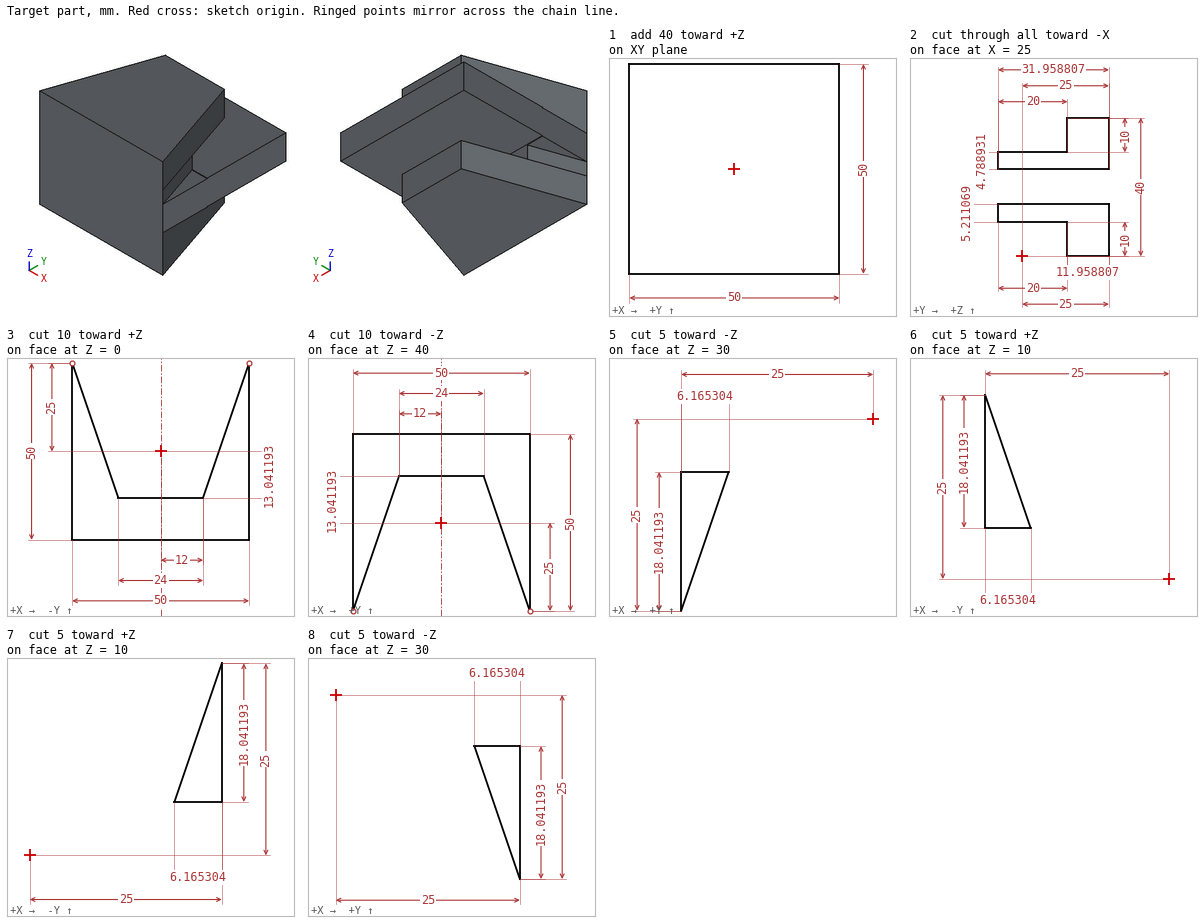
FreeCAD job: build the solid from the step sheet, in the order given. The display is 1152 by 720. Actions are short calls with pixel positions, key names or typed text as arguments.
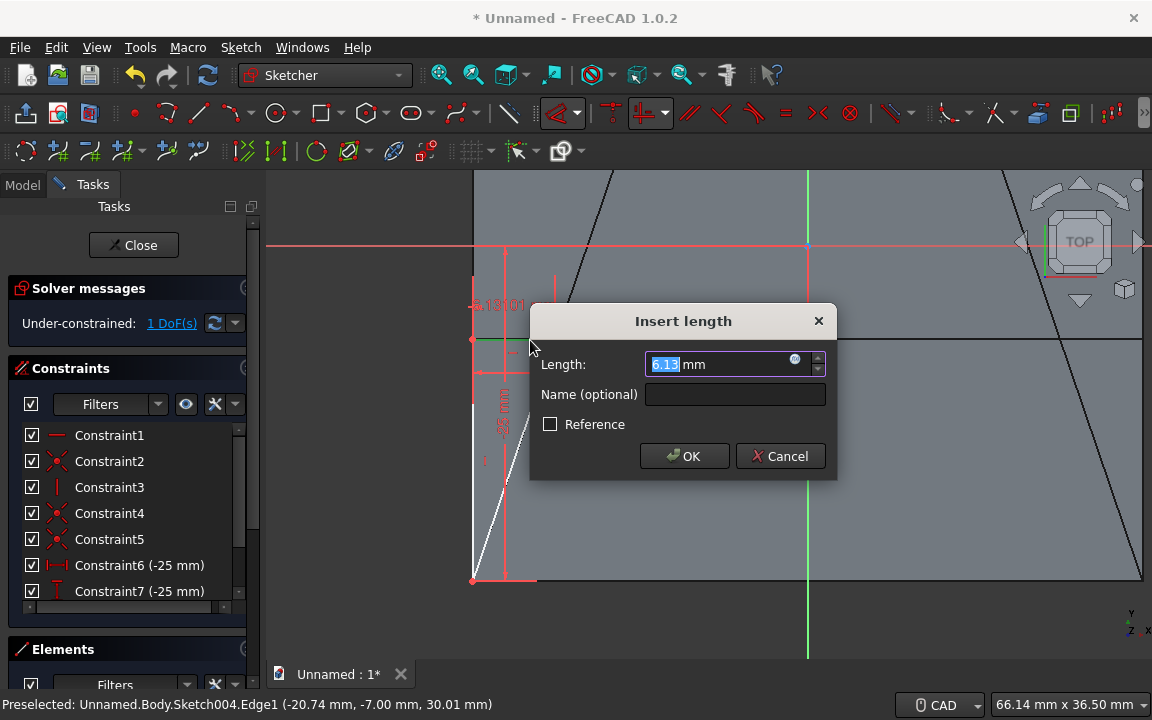
text(6.165304)
key(Return)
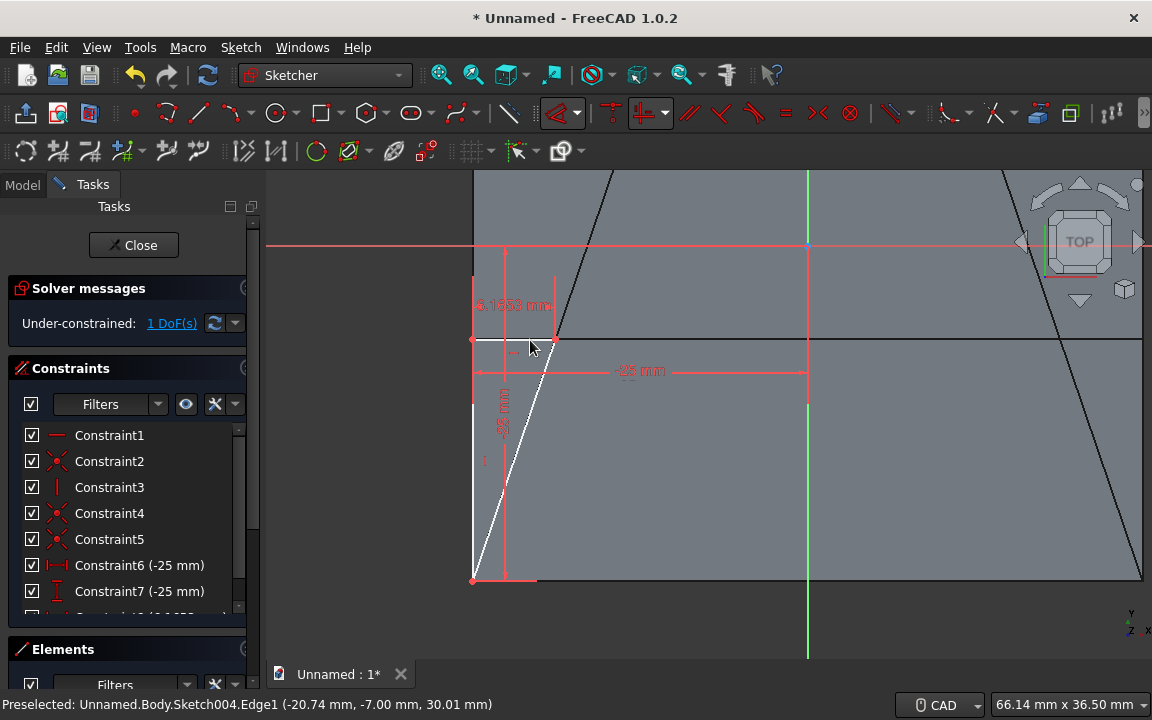
click(473, 412)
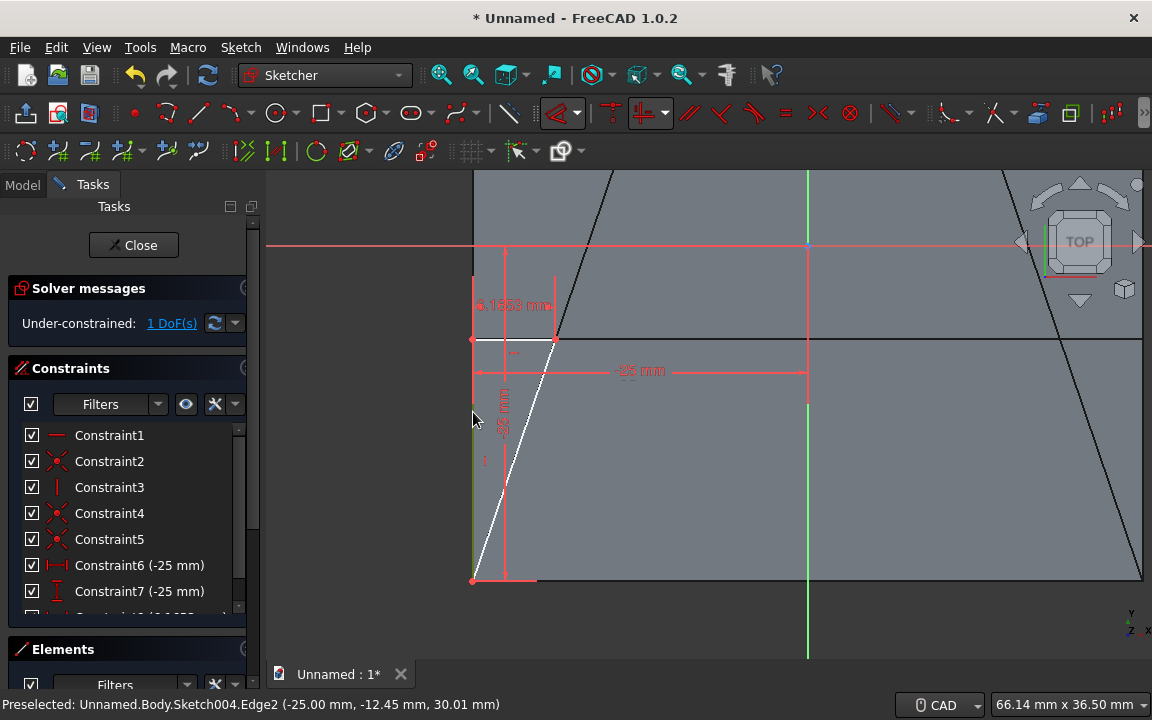
key(i)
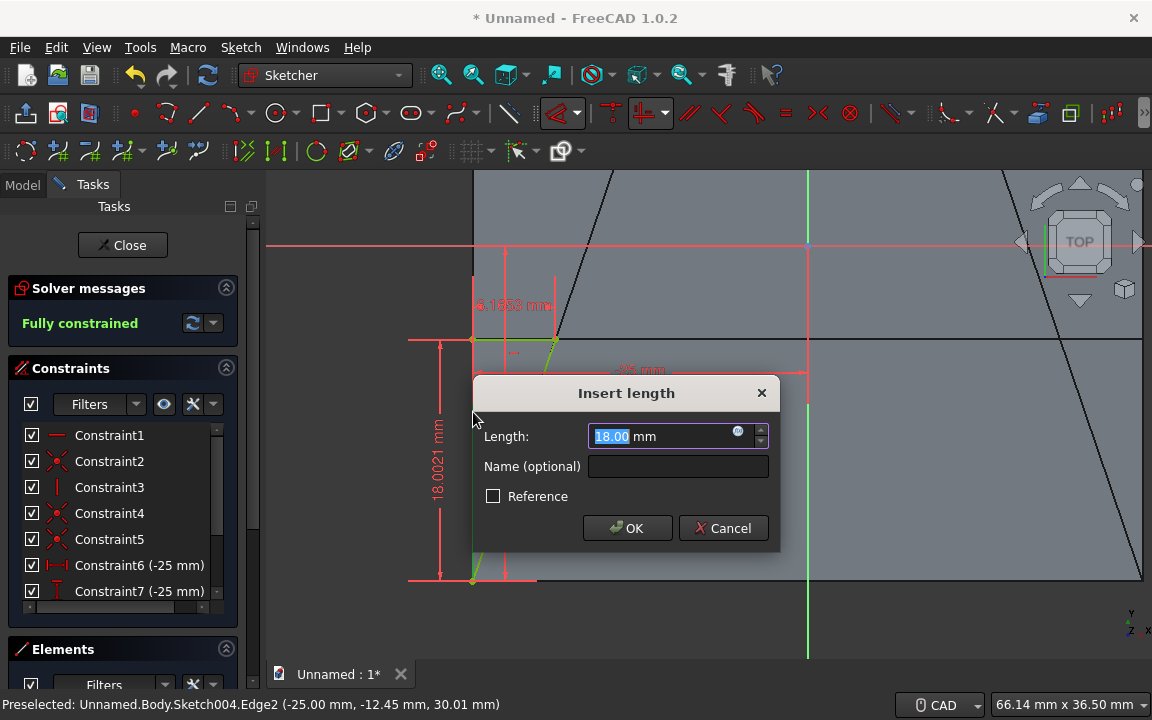
text(18.041193)
key(Return)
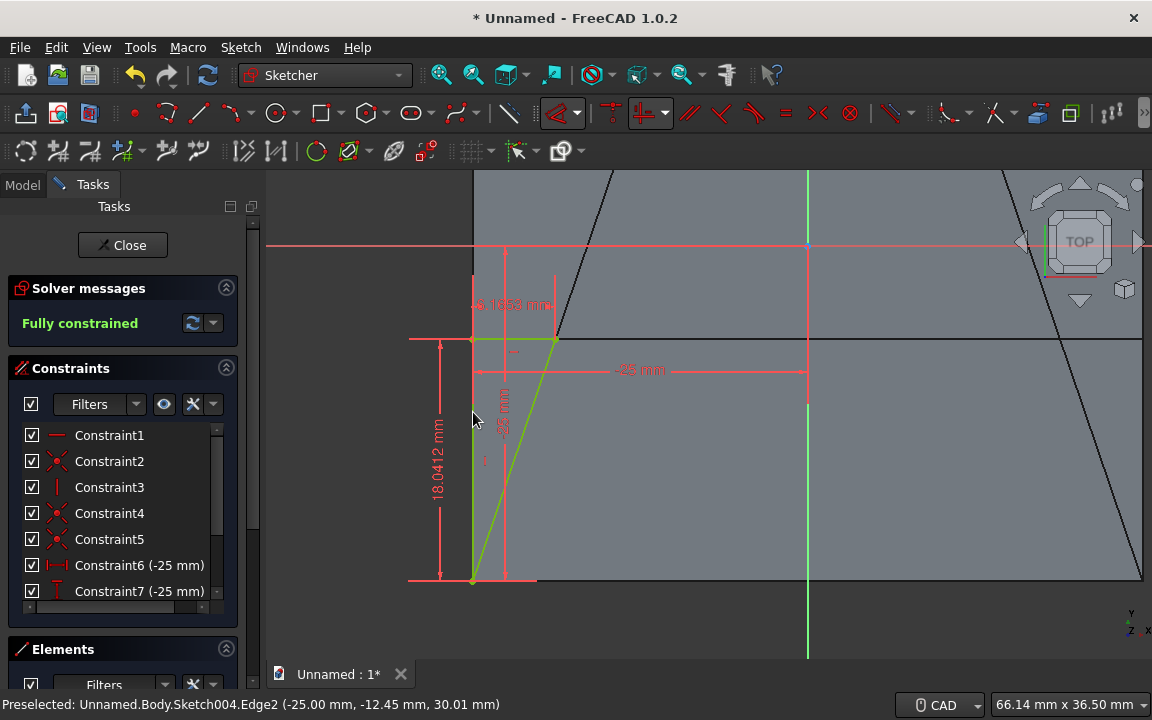
click(123, 245)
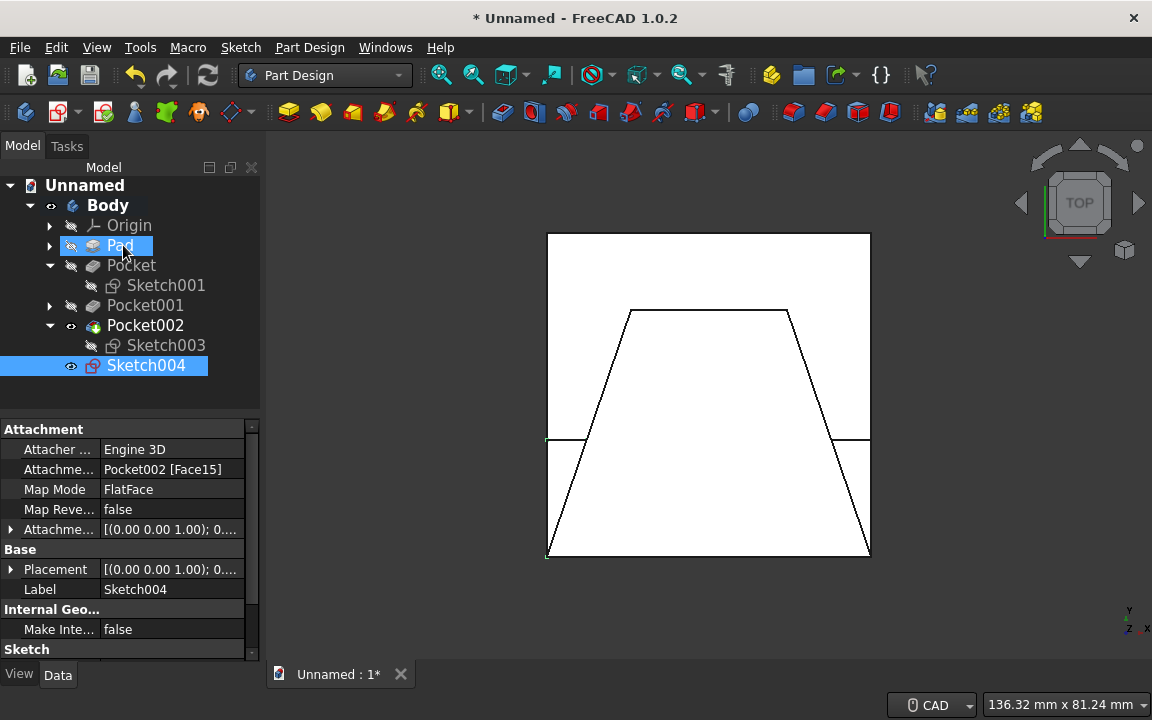
click(504, 112)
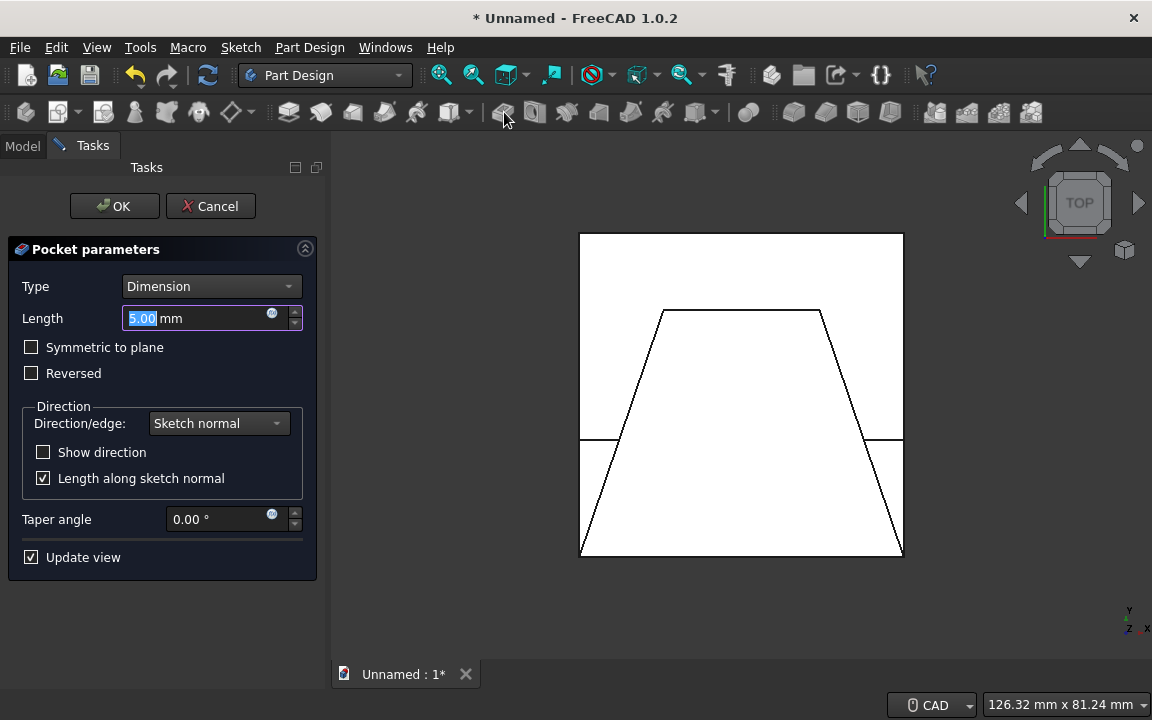
text(5)
key(Tab)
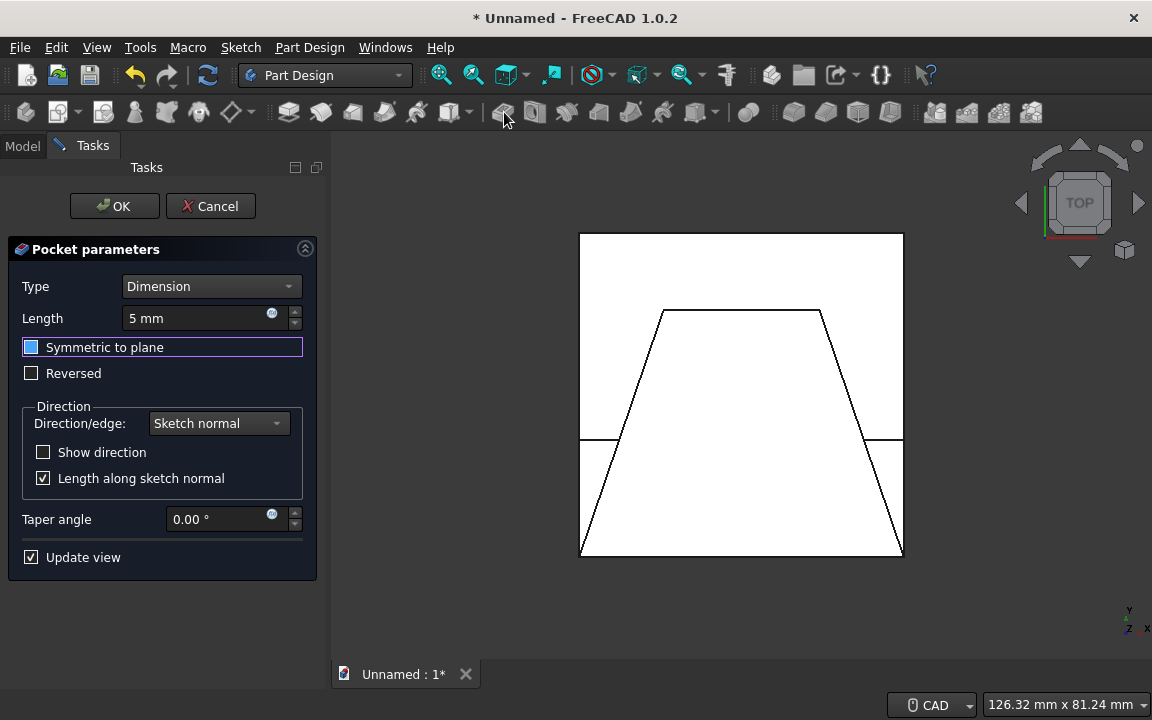
click(115, 206)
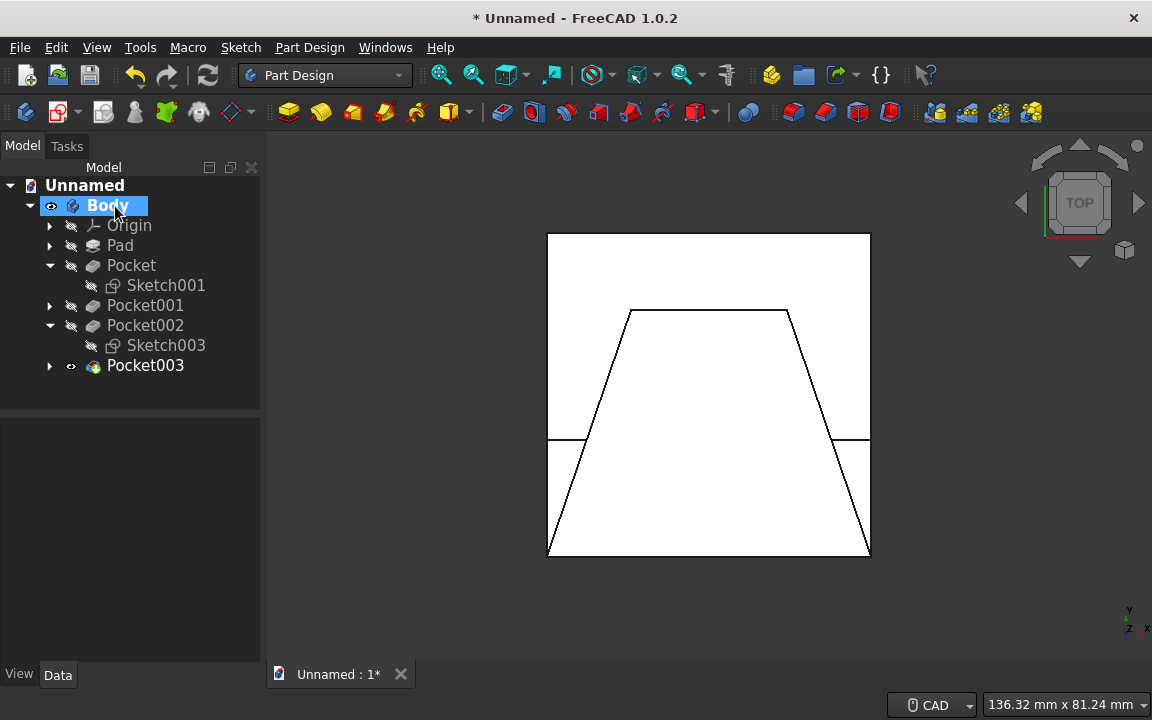
key(5)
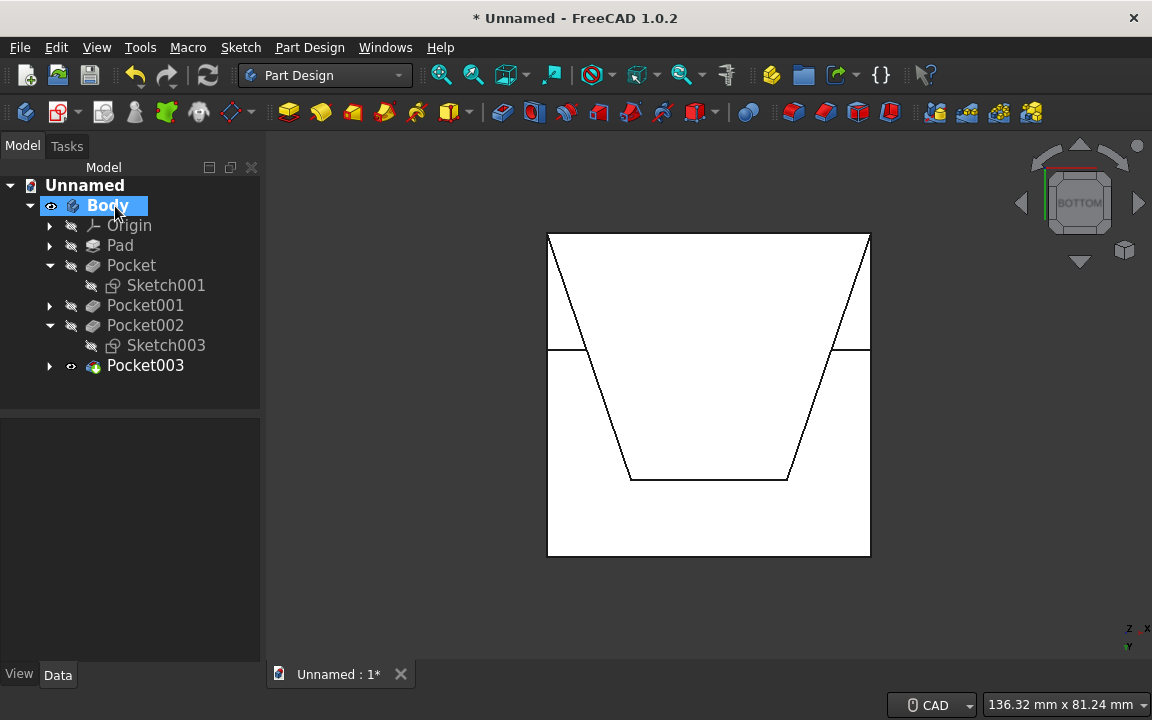
click(857, 324)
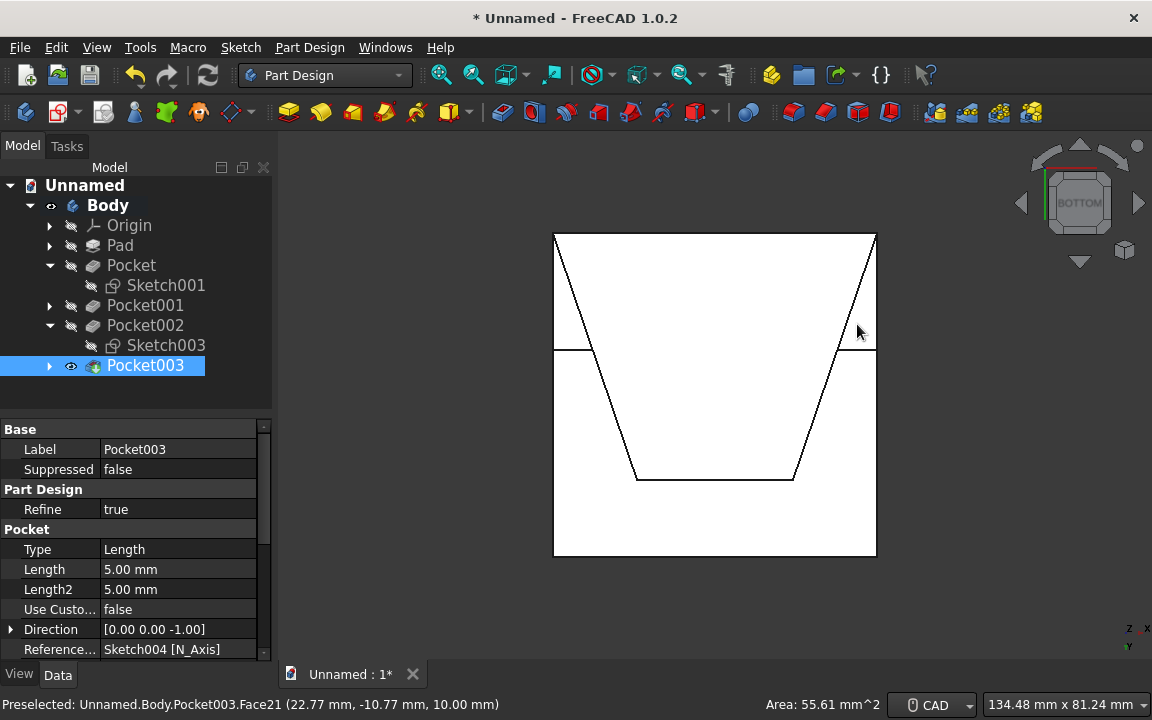
click(58, 112)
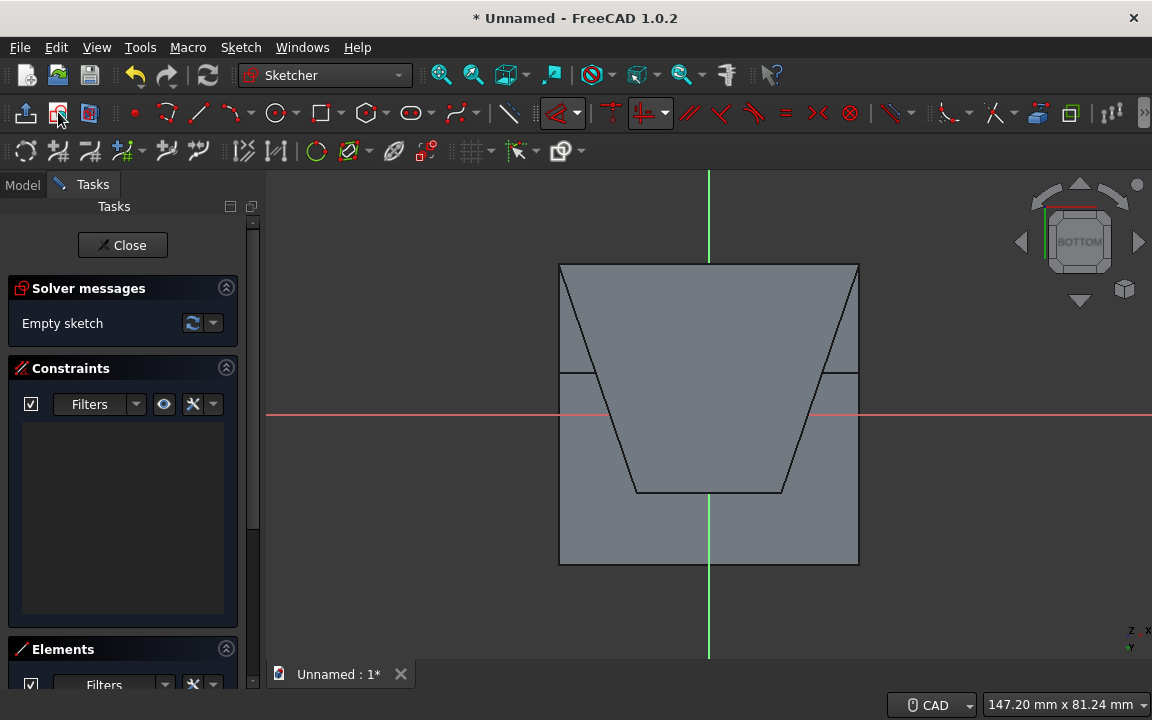
click(90, 114)